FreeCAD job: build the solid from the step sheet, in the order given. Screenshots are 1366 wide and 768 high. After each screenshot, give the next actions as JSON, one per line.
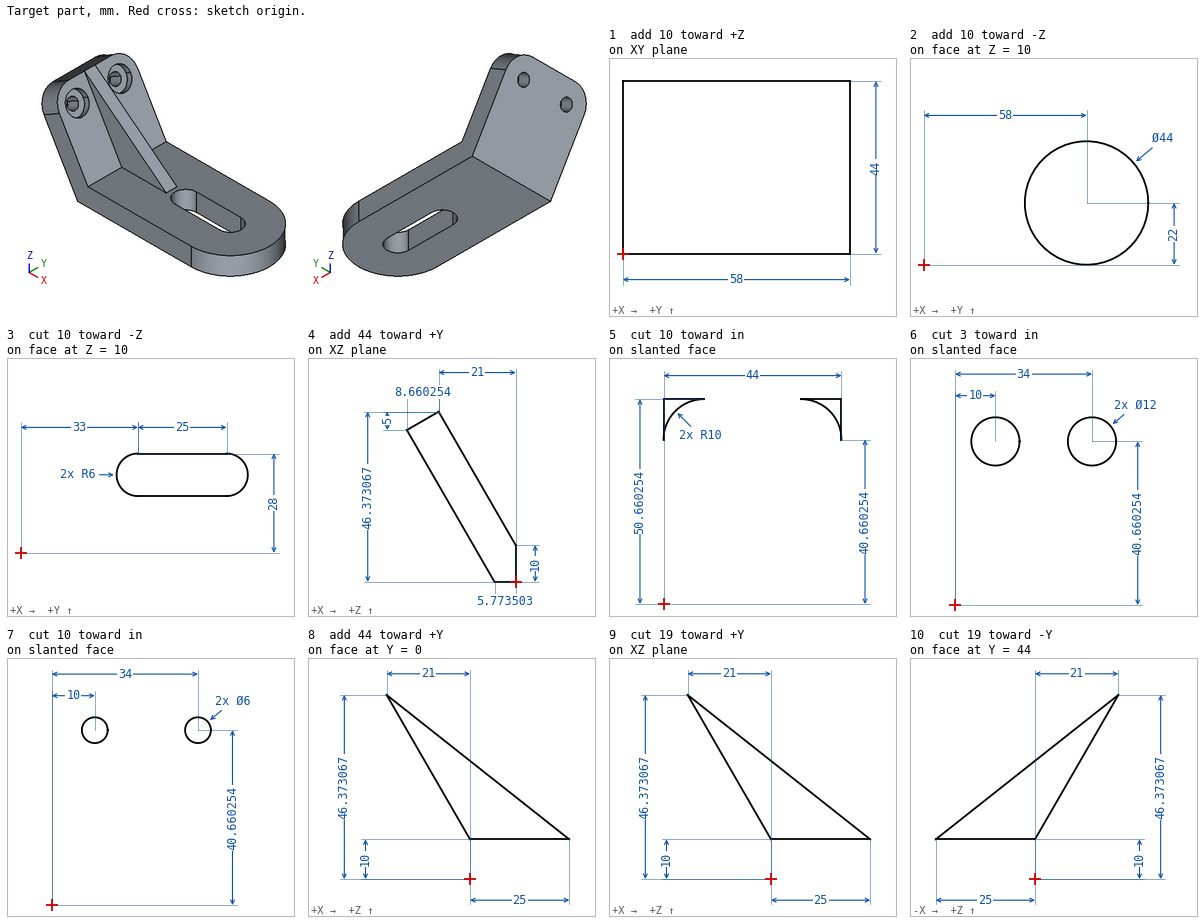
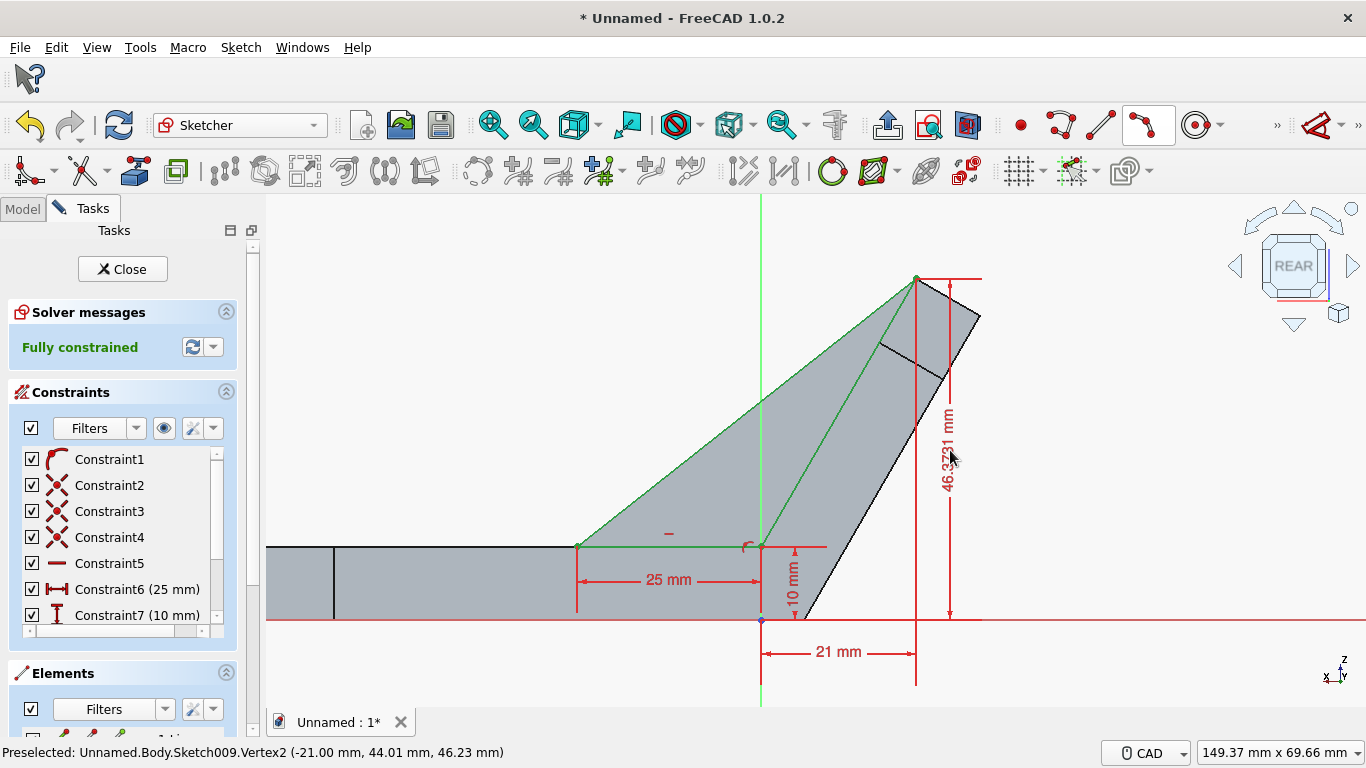
{"action": "left_click", "coordinate": [123, 269]}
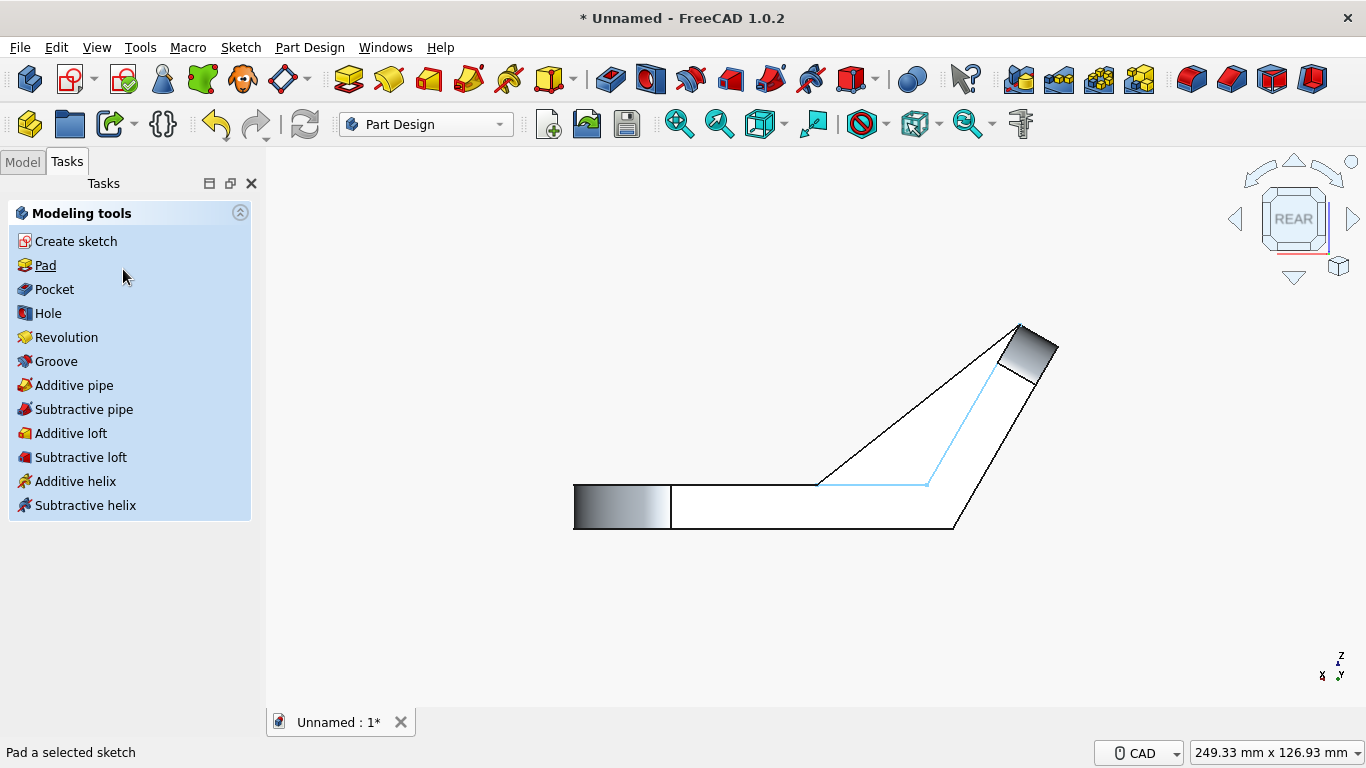
{"action": "left_click", "coordinate": [612, 80]}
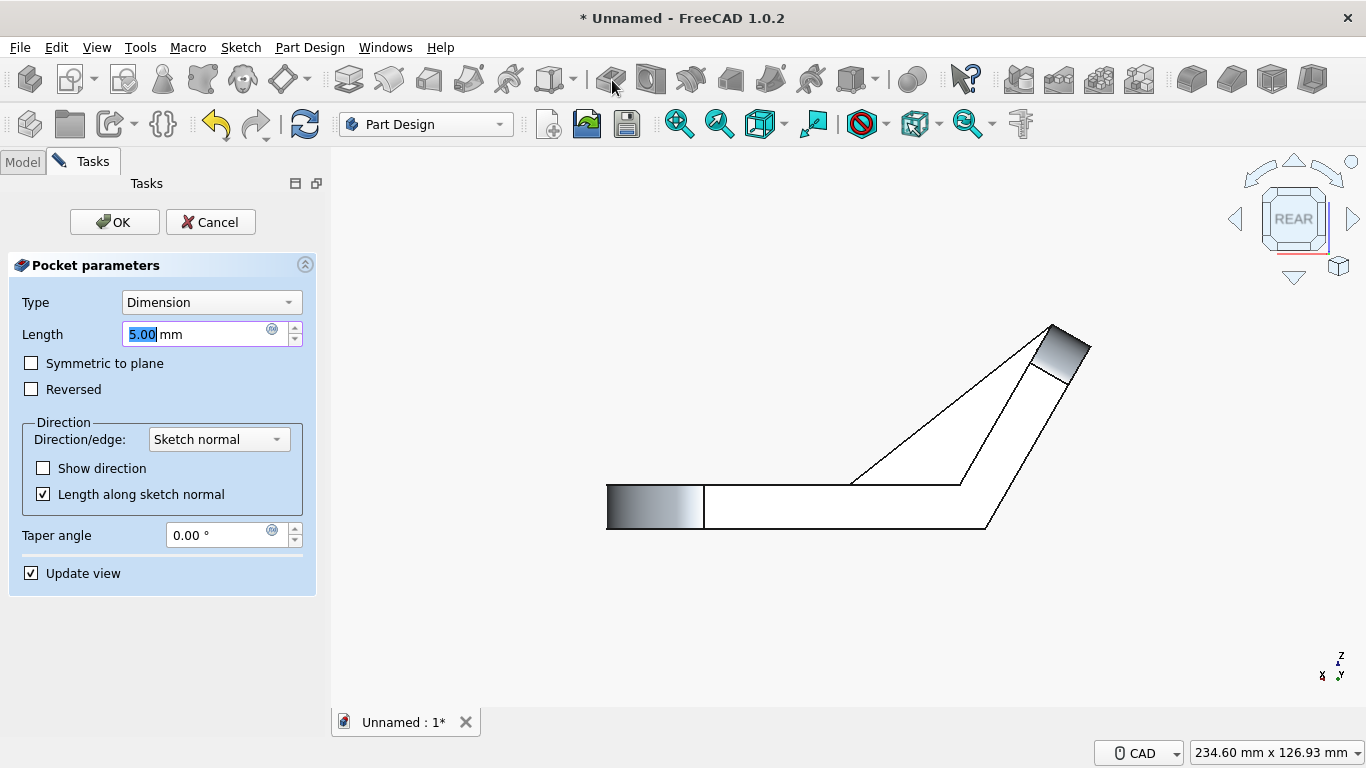
{"action": "type", "text": "19"}
{"action": "key", "text": "Tab"}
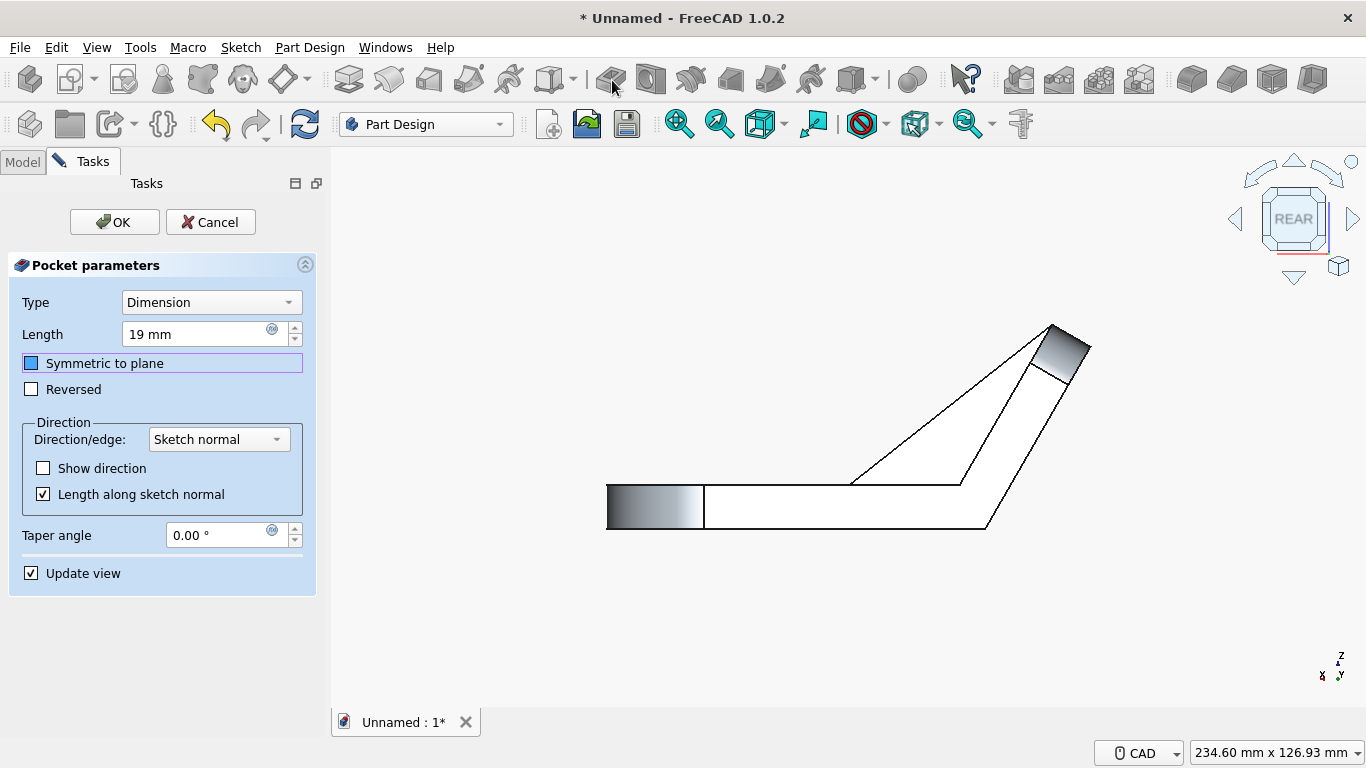
{"action": "left_click", "coordinate": [115, 222]}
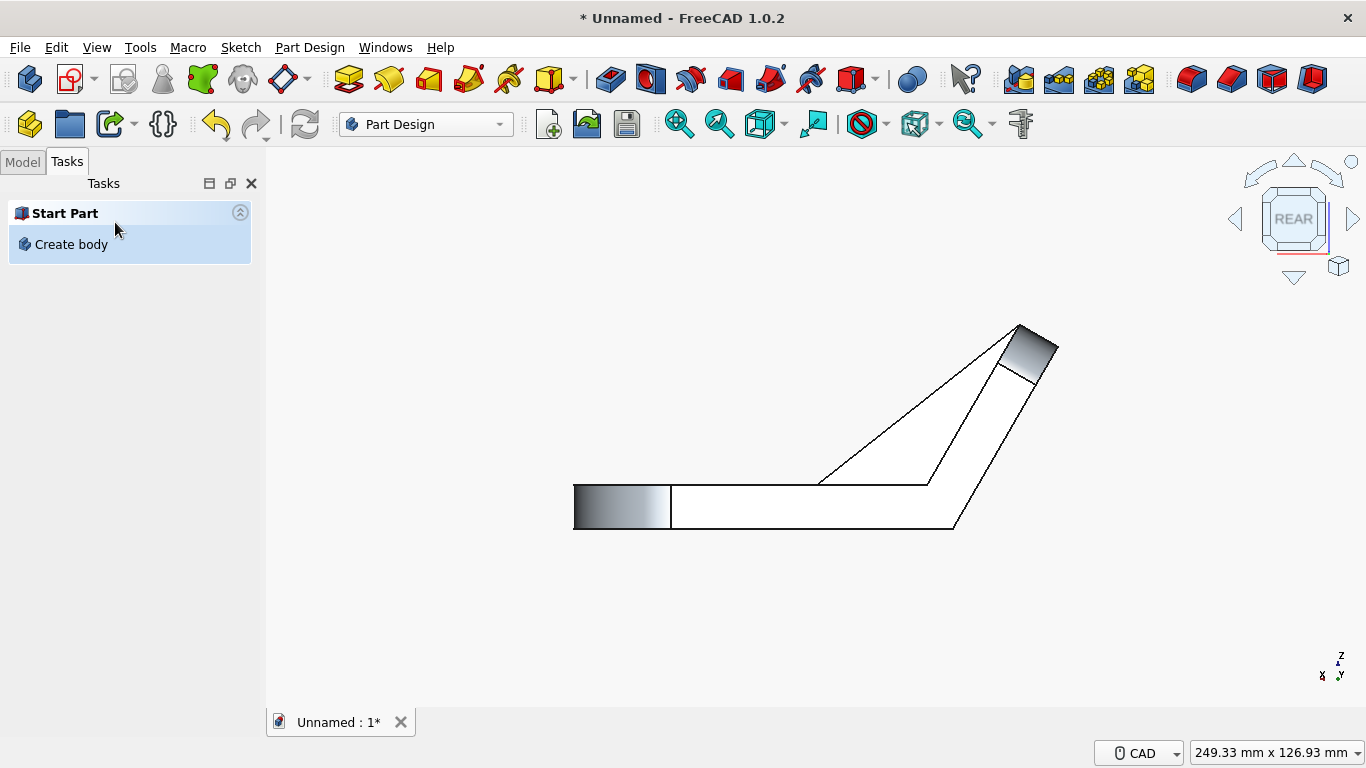
{"action": "key", "text": "0"}